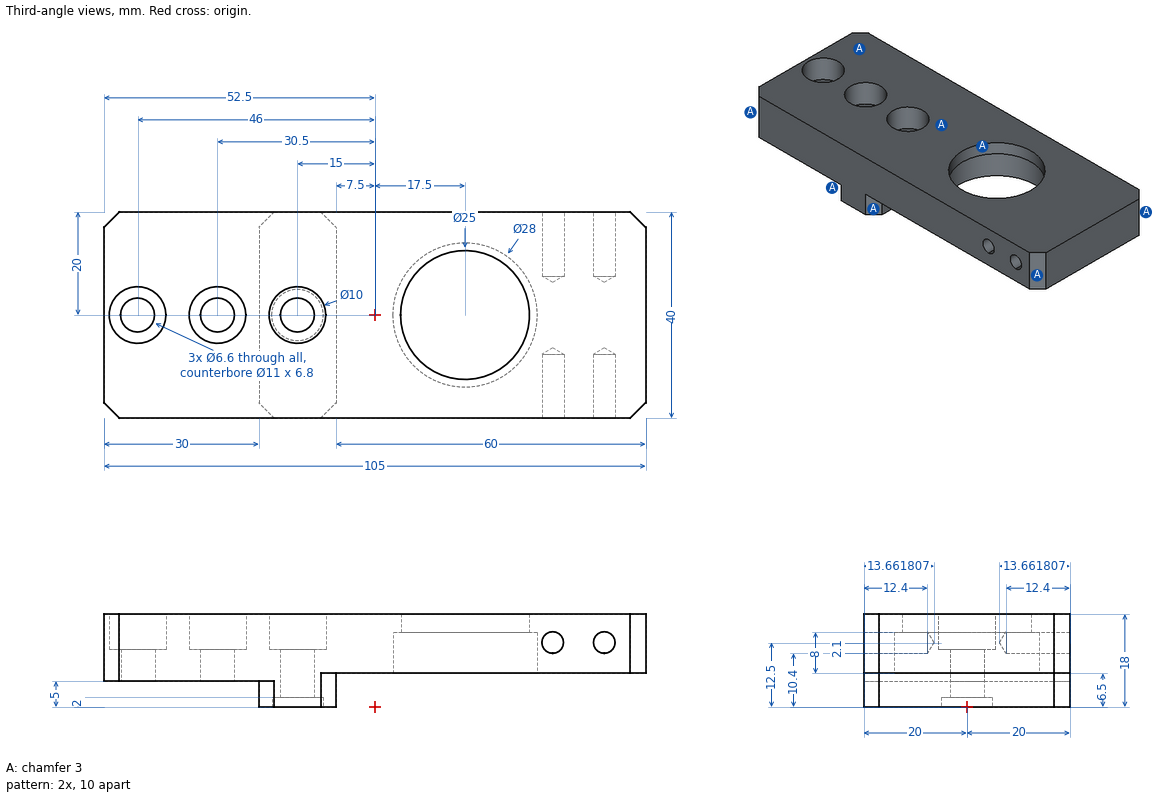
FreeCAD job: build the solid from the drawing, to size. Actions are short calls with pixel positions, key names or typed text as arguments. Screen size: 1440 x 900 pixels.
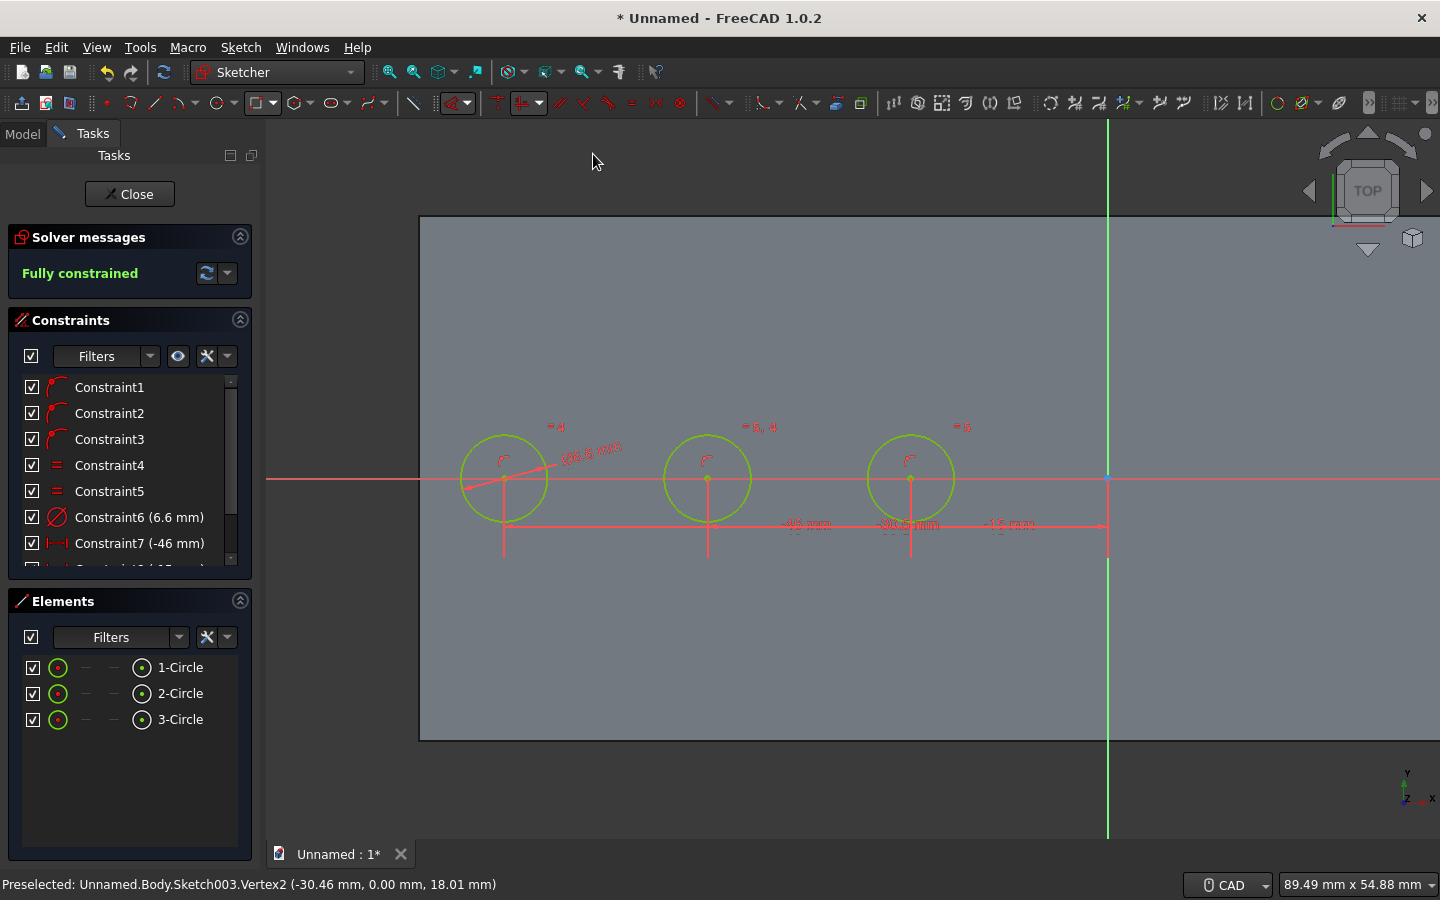
click(130, 194)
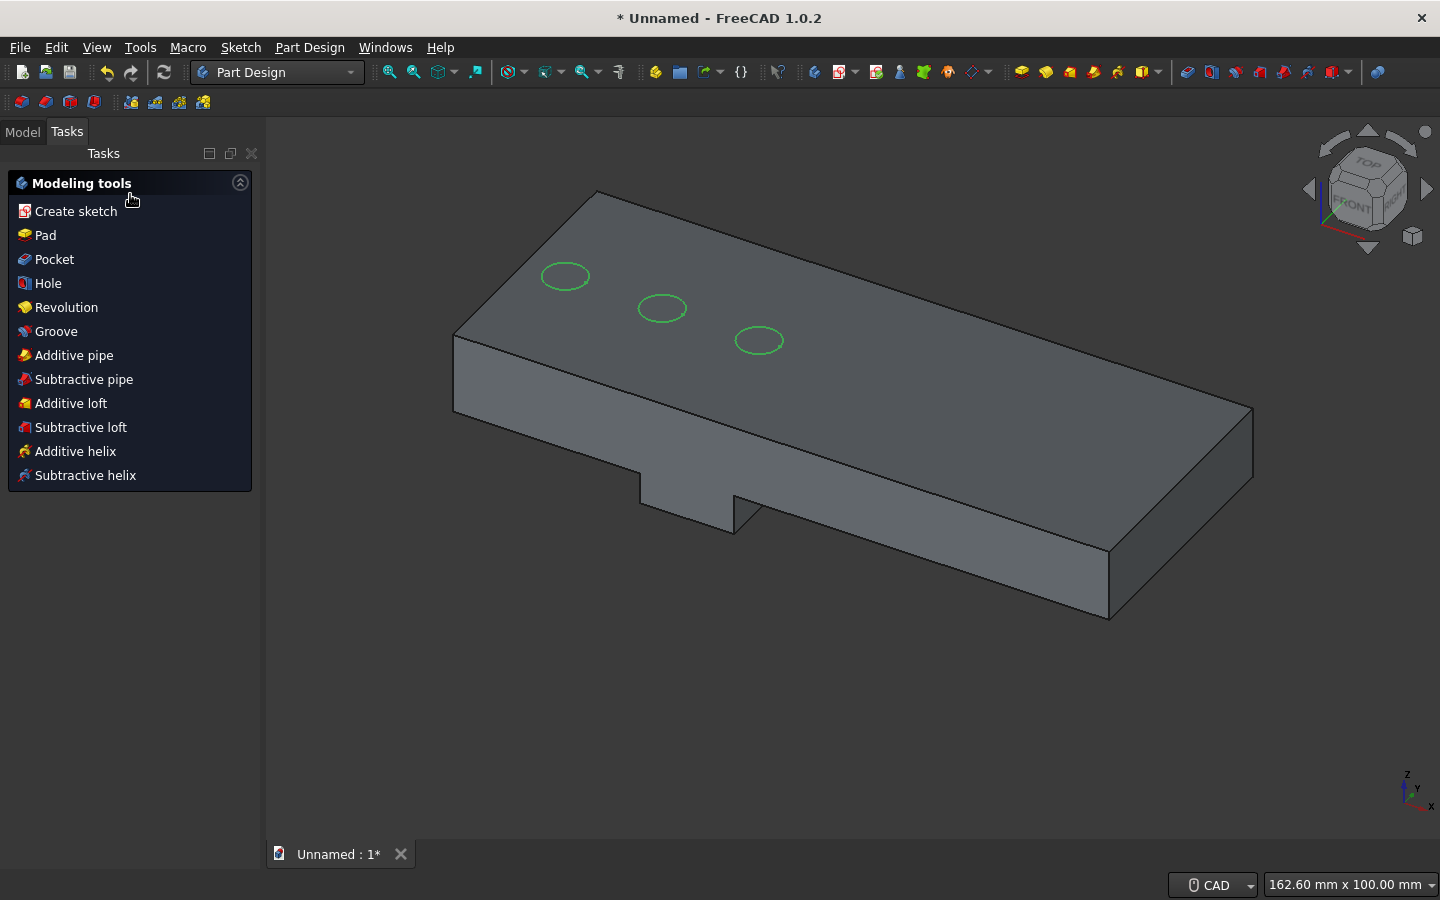
click(1212, 72)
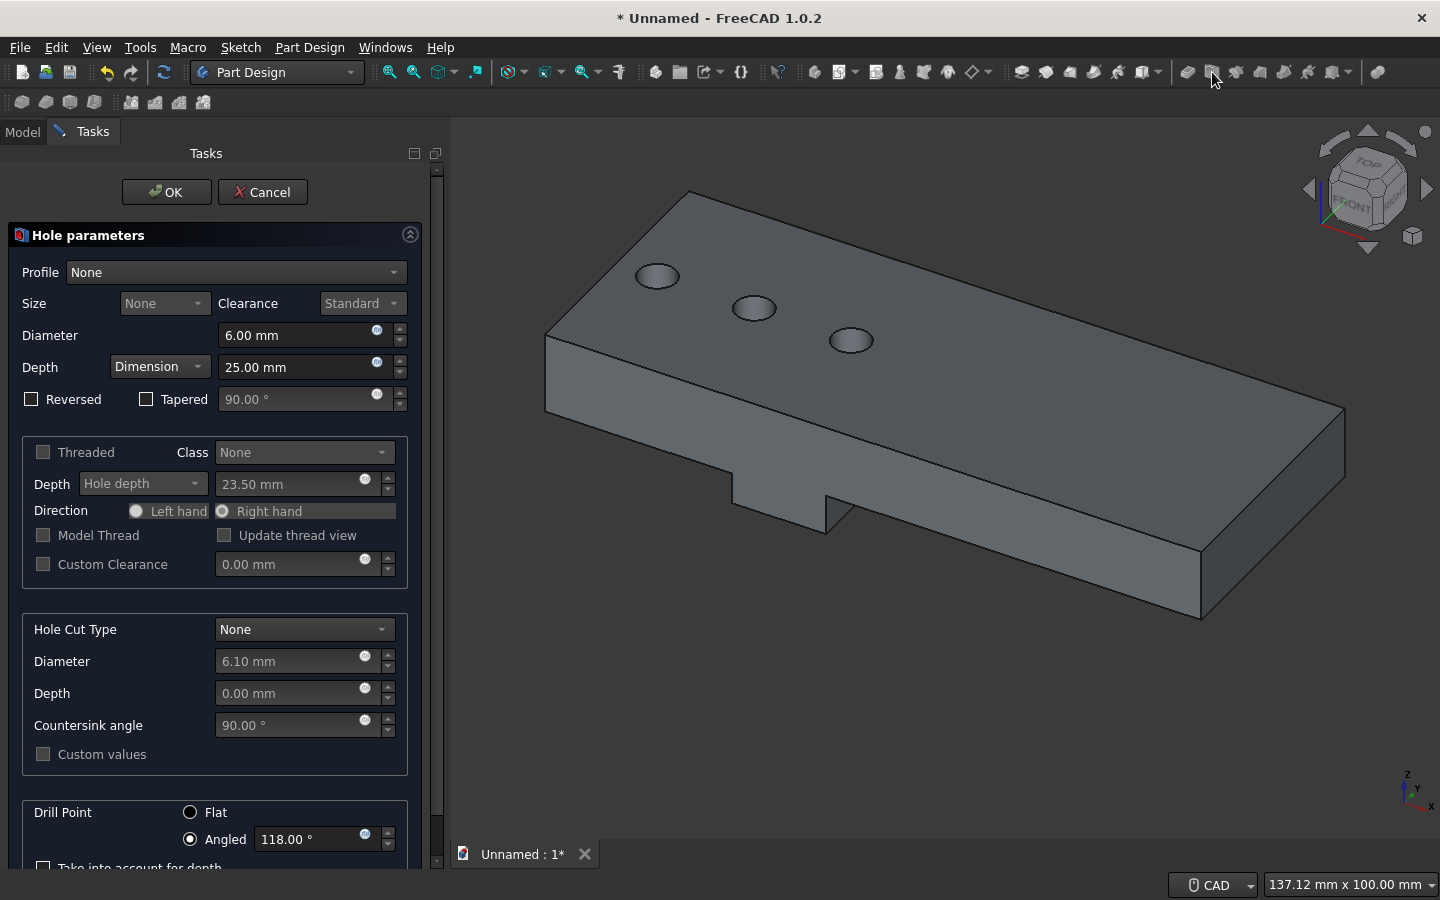
triple_click(305, 335)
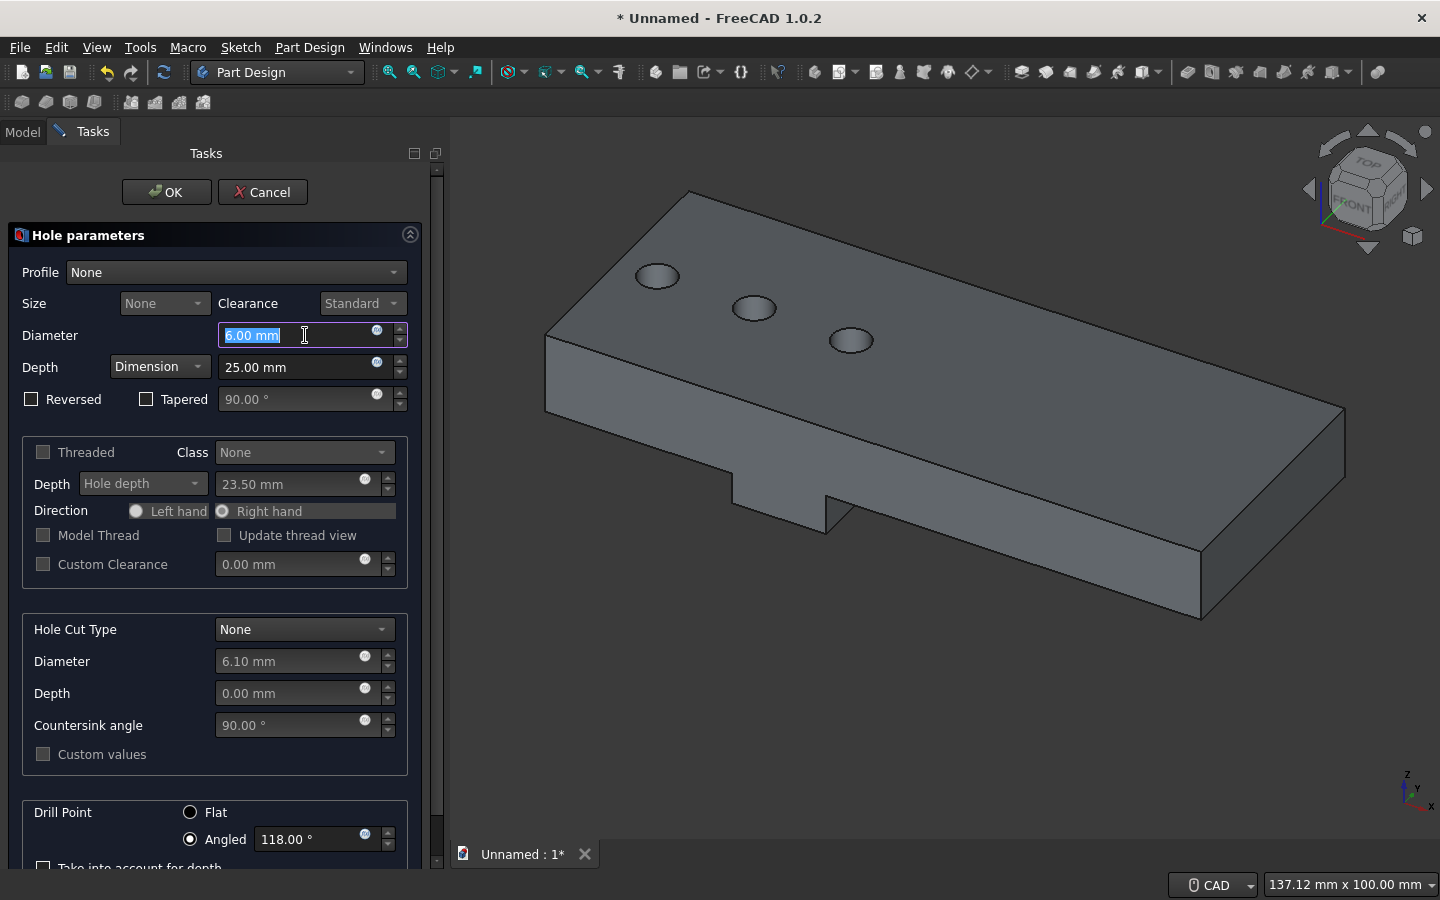
text(6.6)
key(Tab)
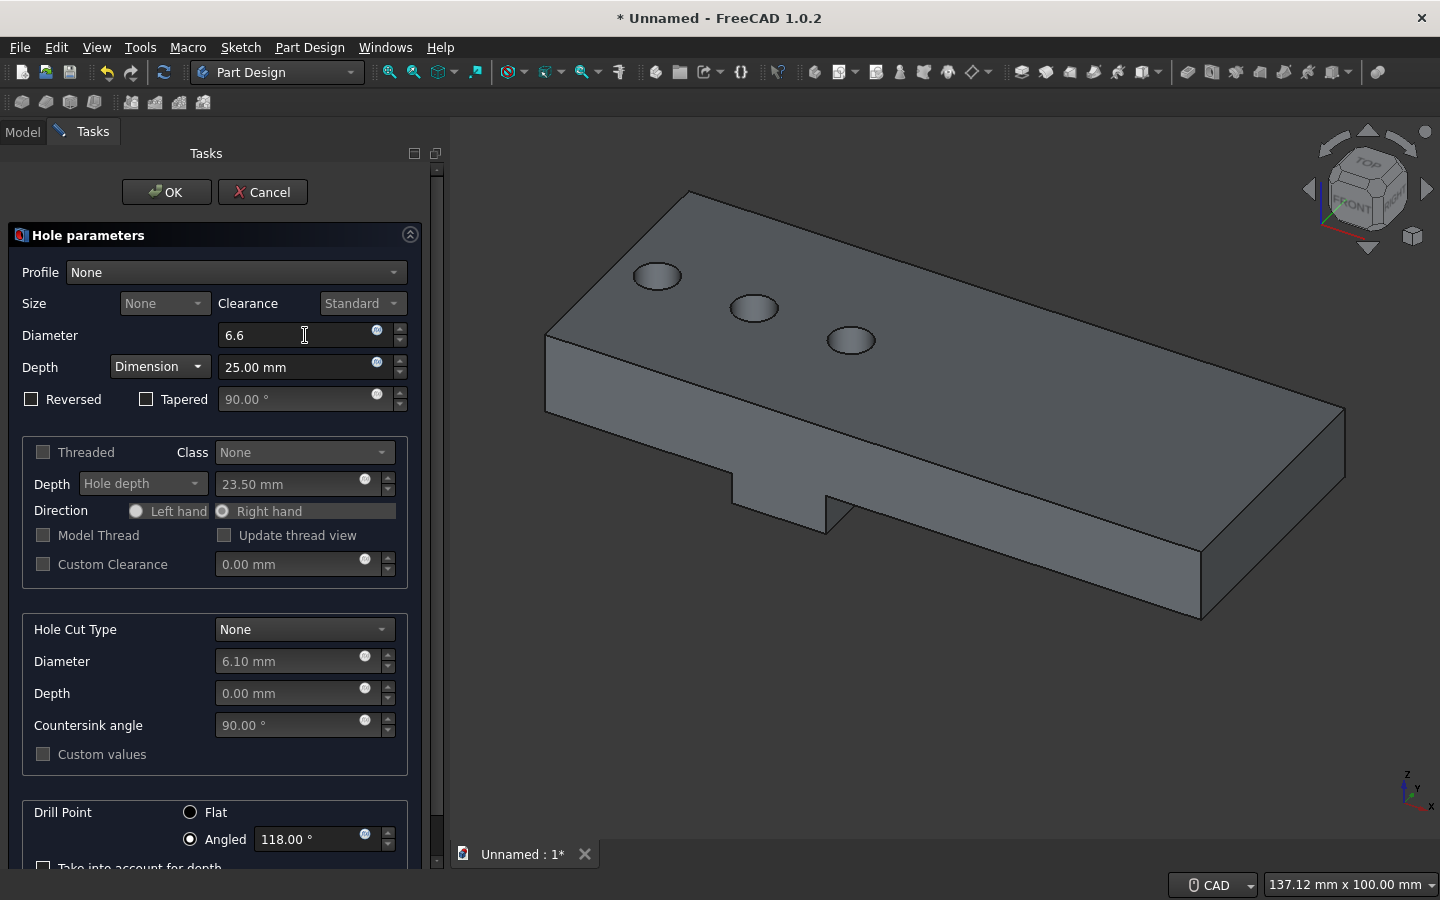
click(161, 366)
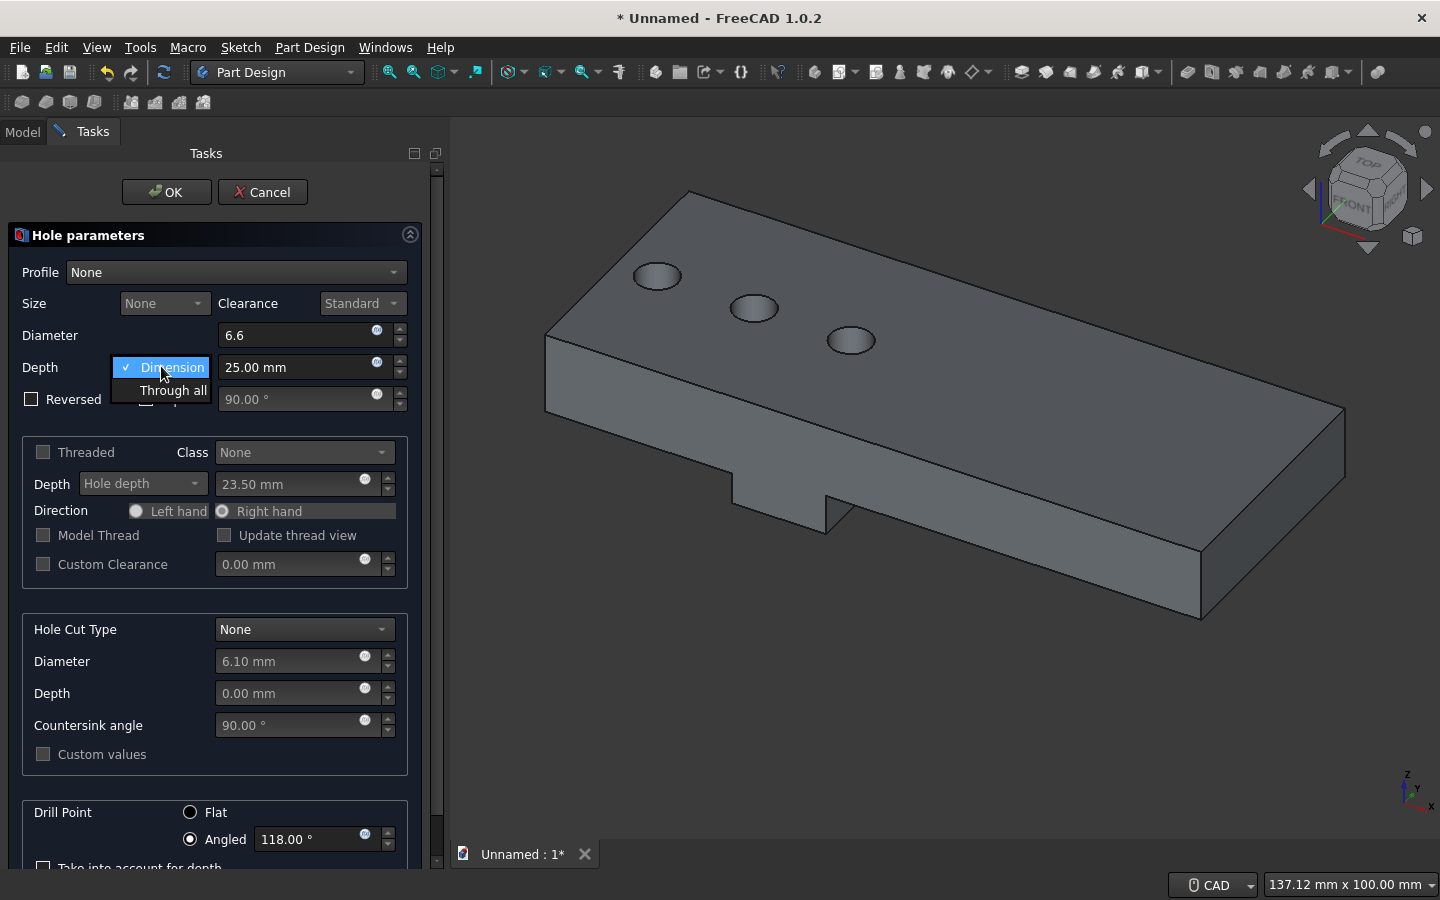
click(160, 390)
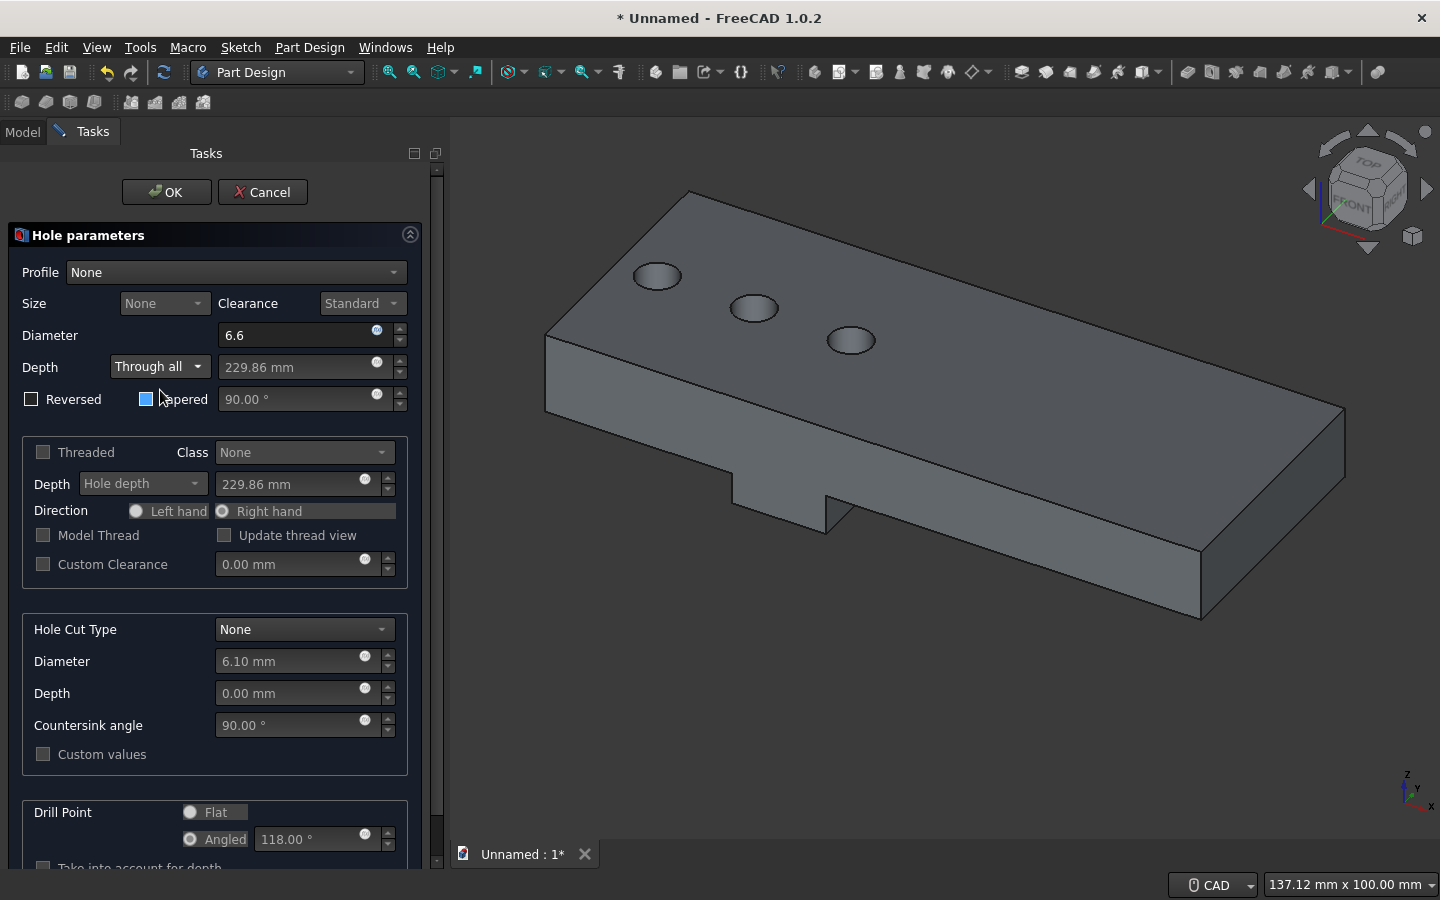
click(306, 630)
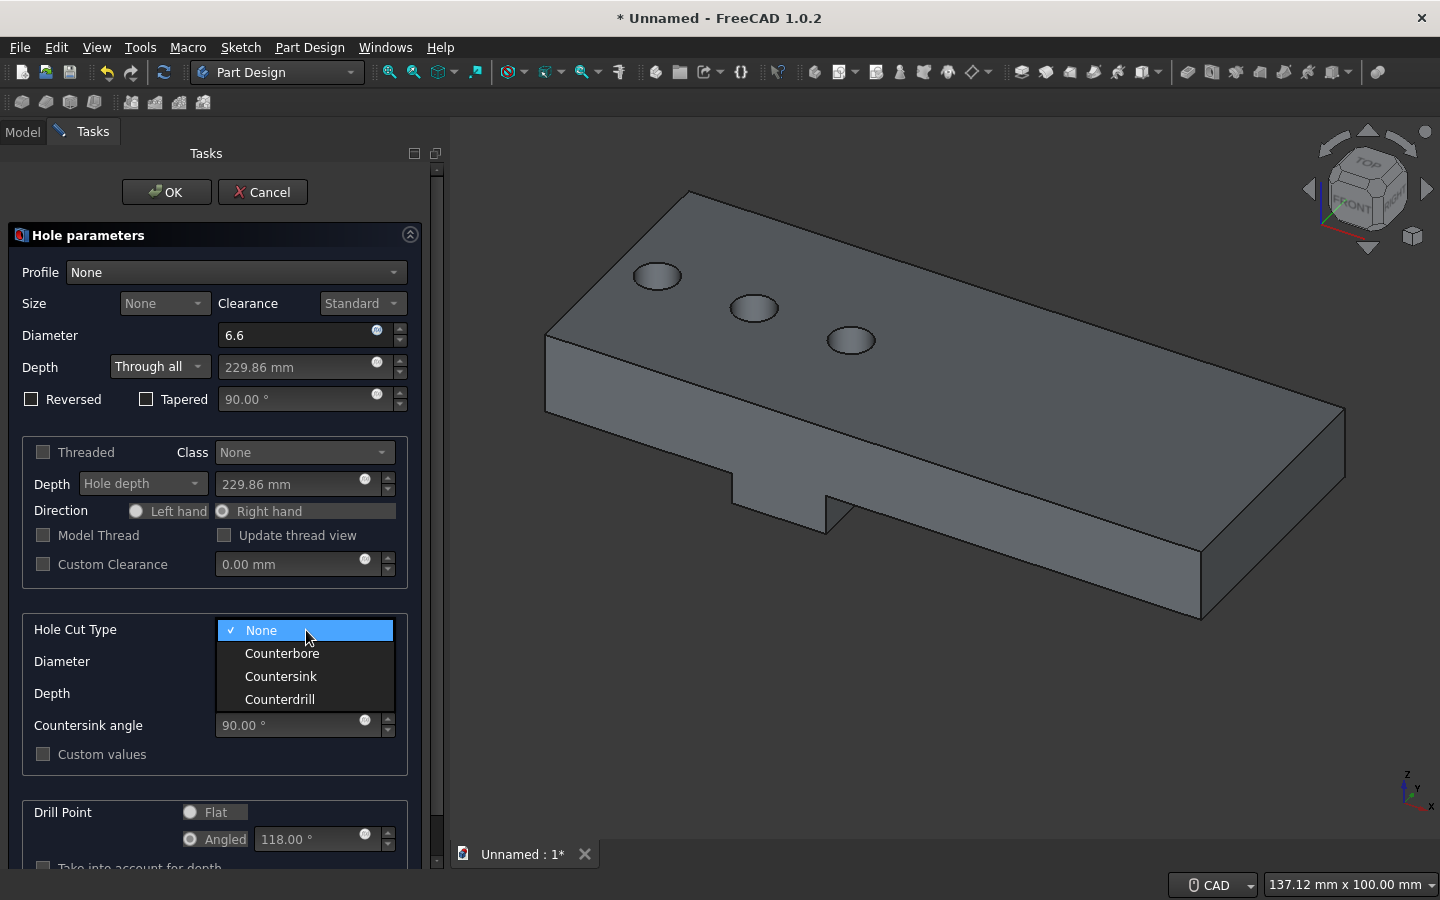
click(304, 654)